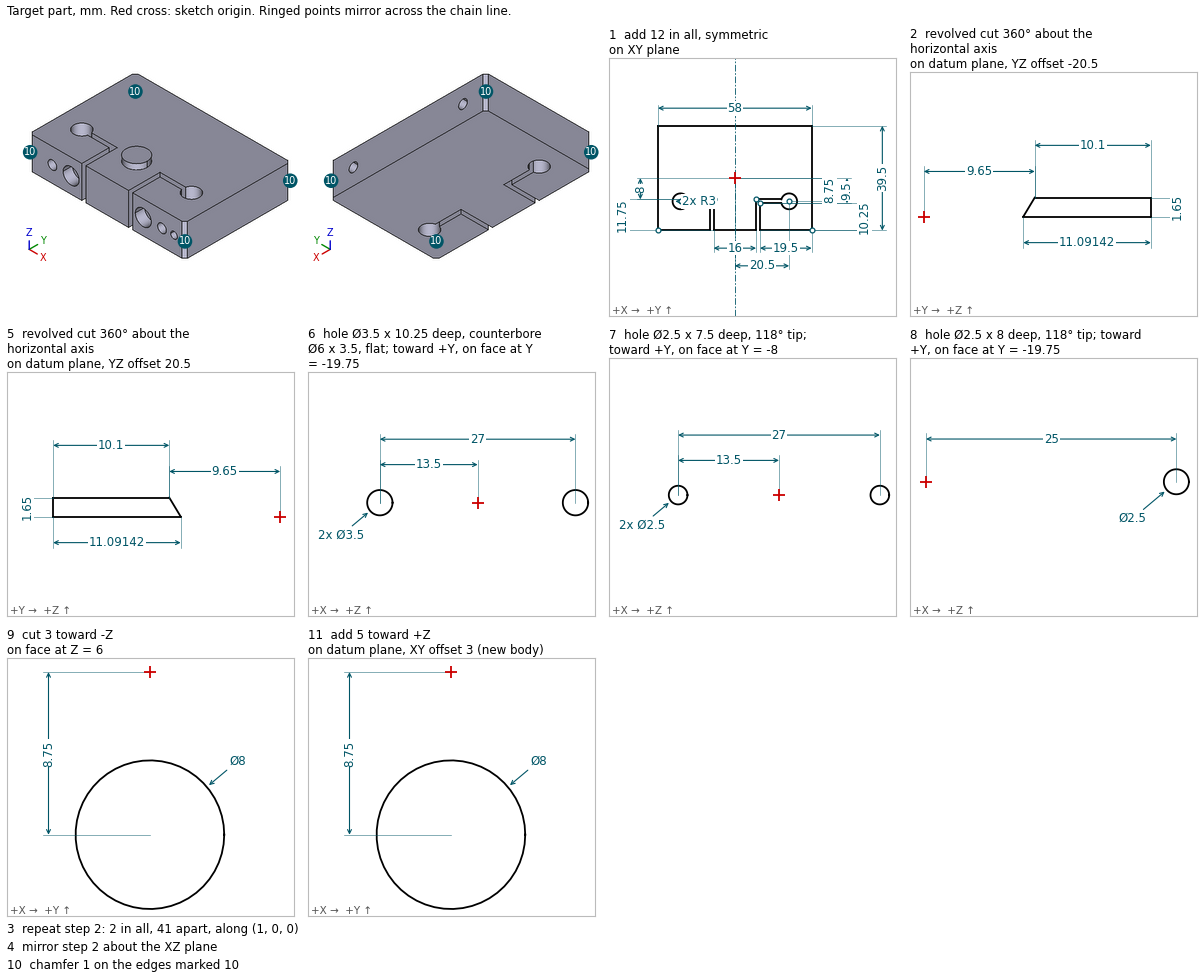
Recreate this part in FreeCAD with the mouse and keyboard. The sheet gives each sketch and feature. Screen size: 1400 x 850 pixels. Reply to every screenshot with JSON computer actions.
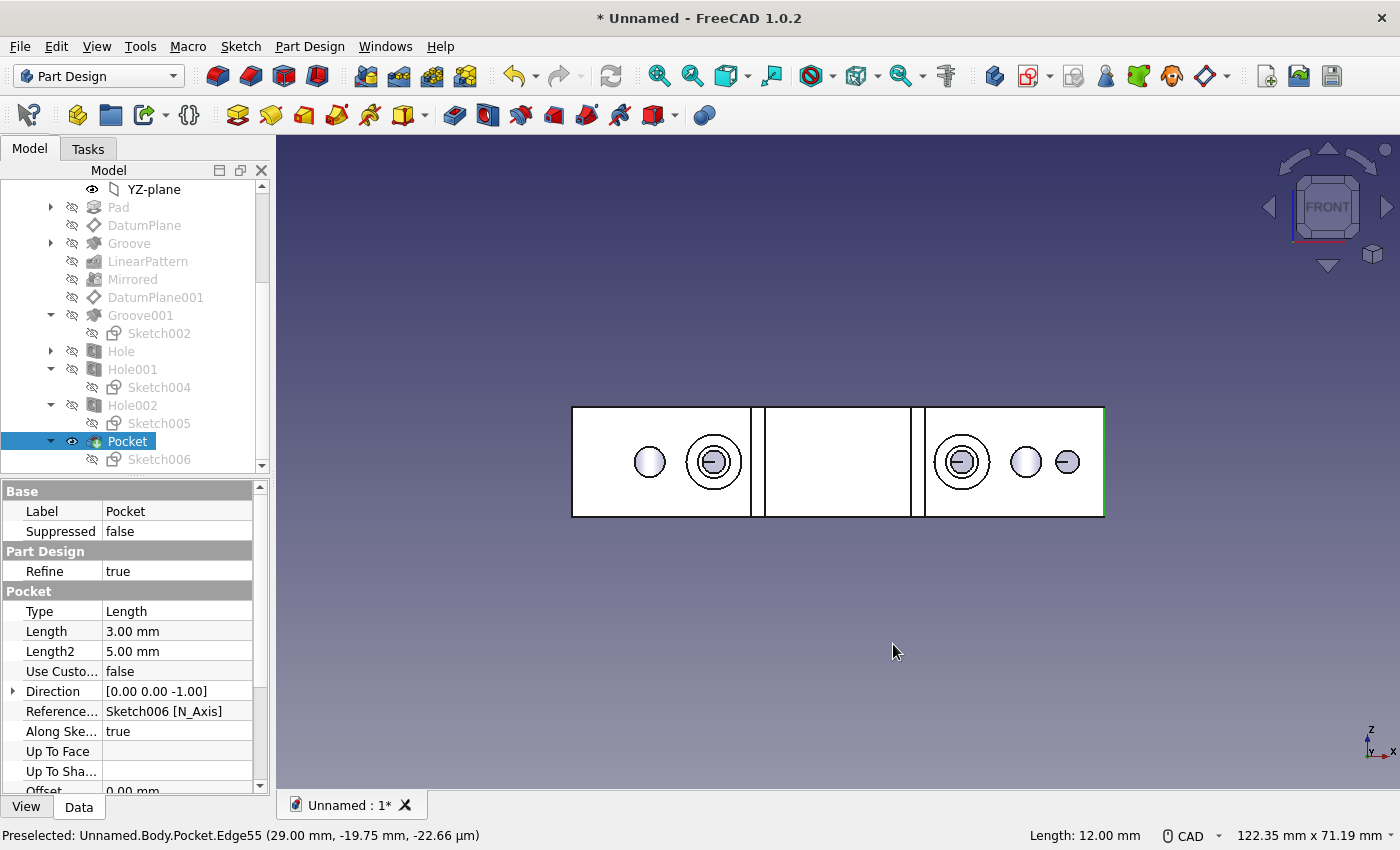
{"action": "left_click", "coordinate": [572, 461], "text": "ctrl"}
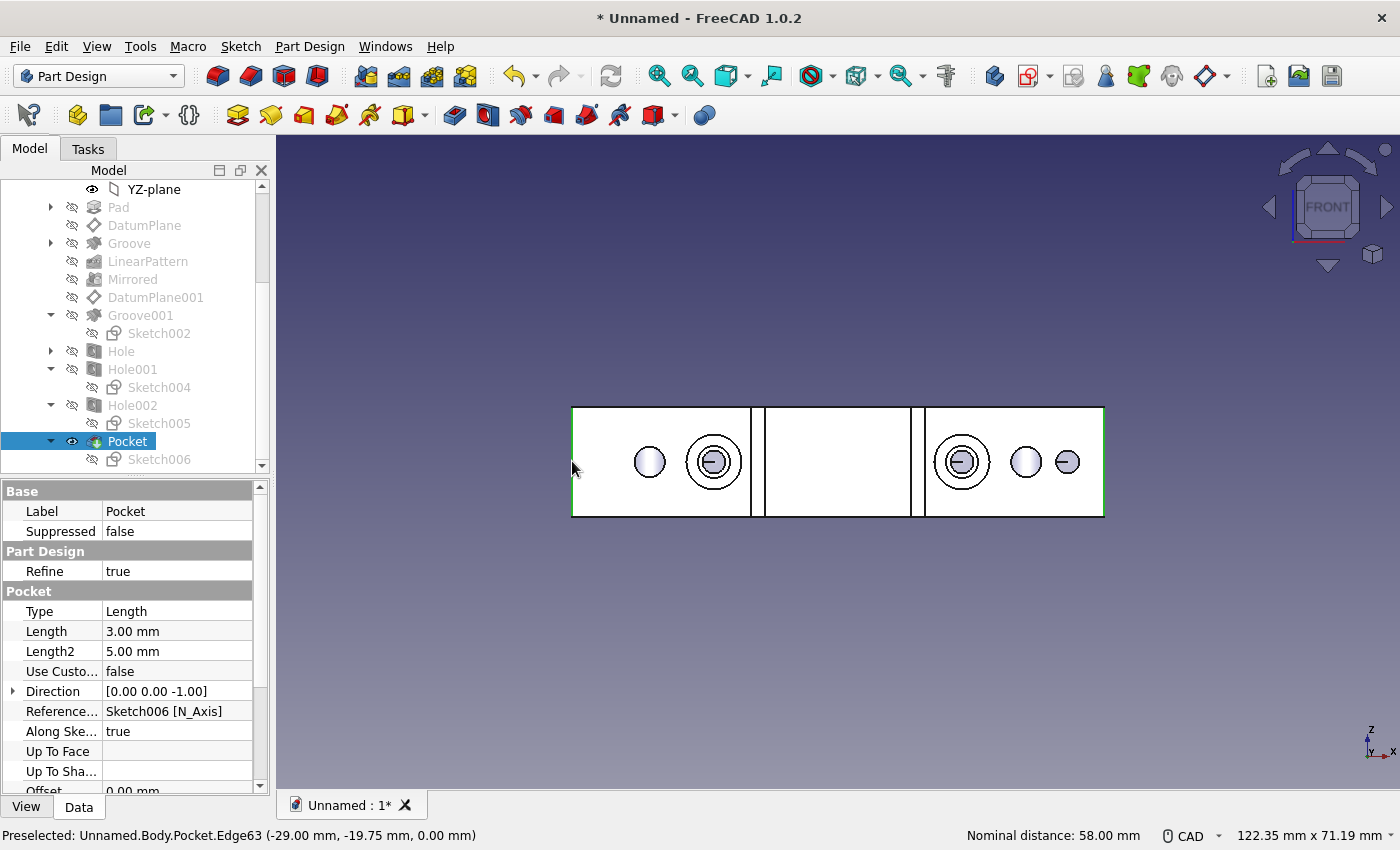
{"action": "key", "text": "3"}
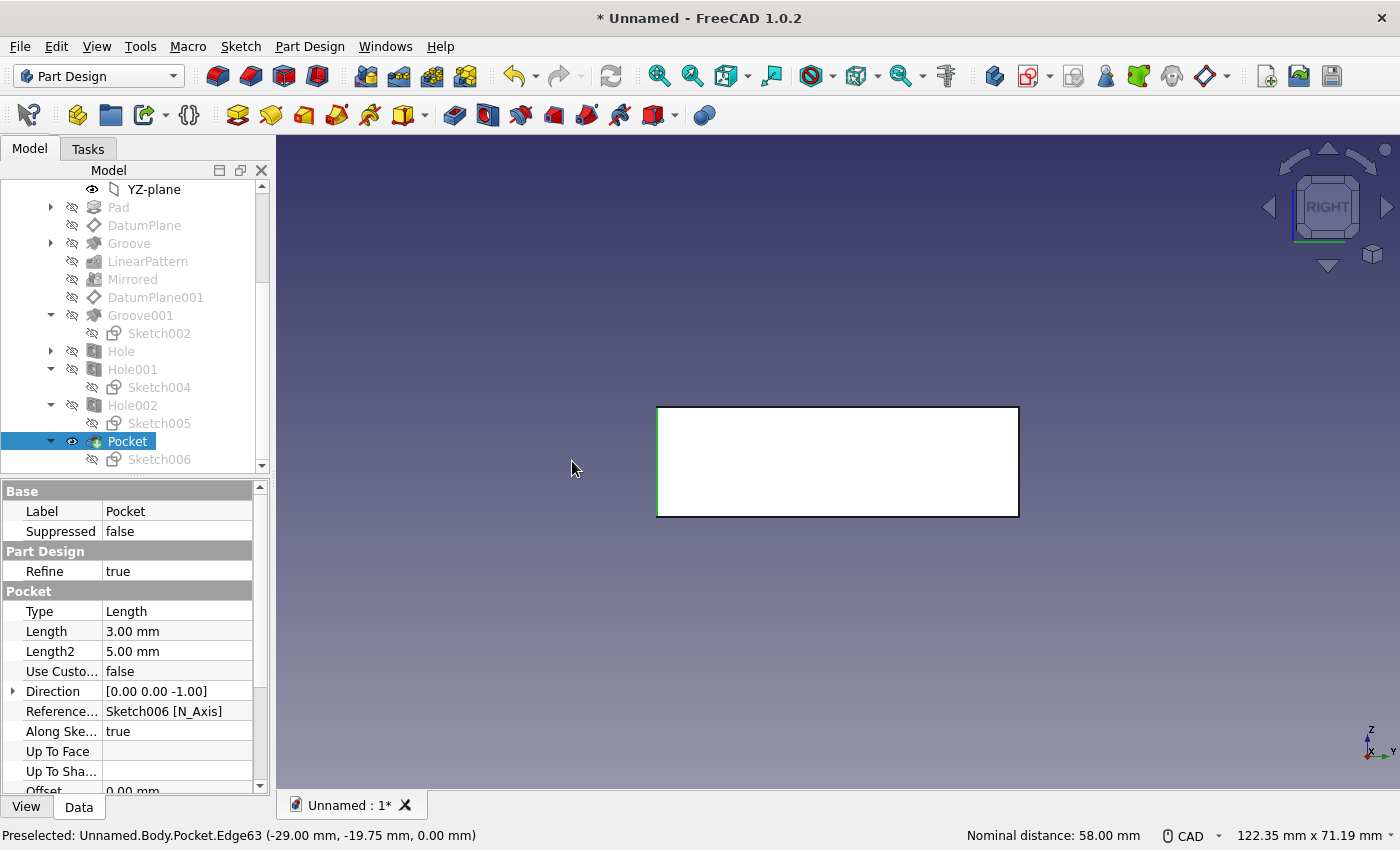
{"action": "left_click", "coordinate": [660, 76]}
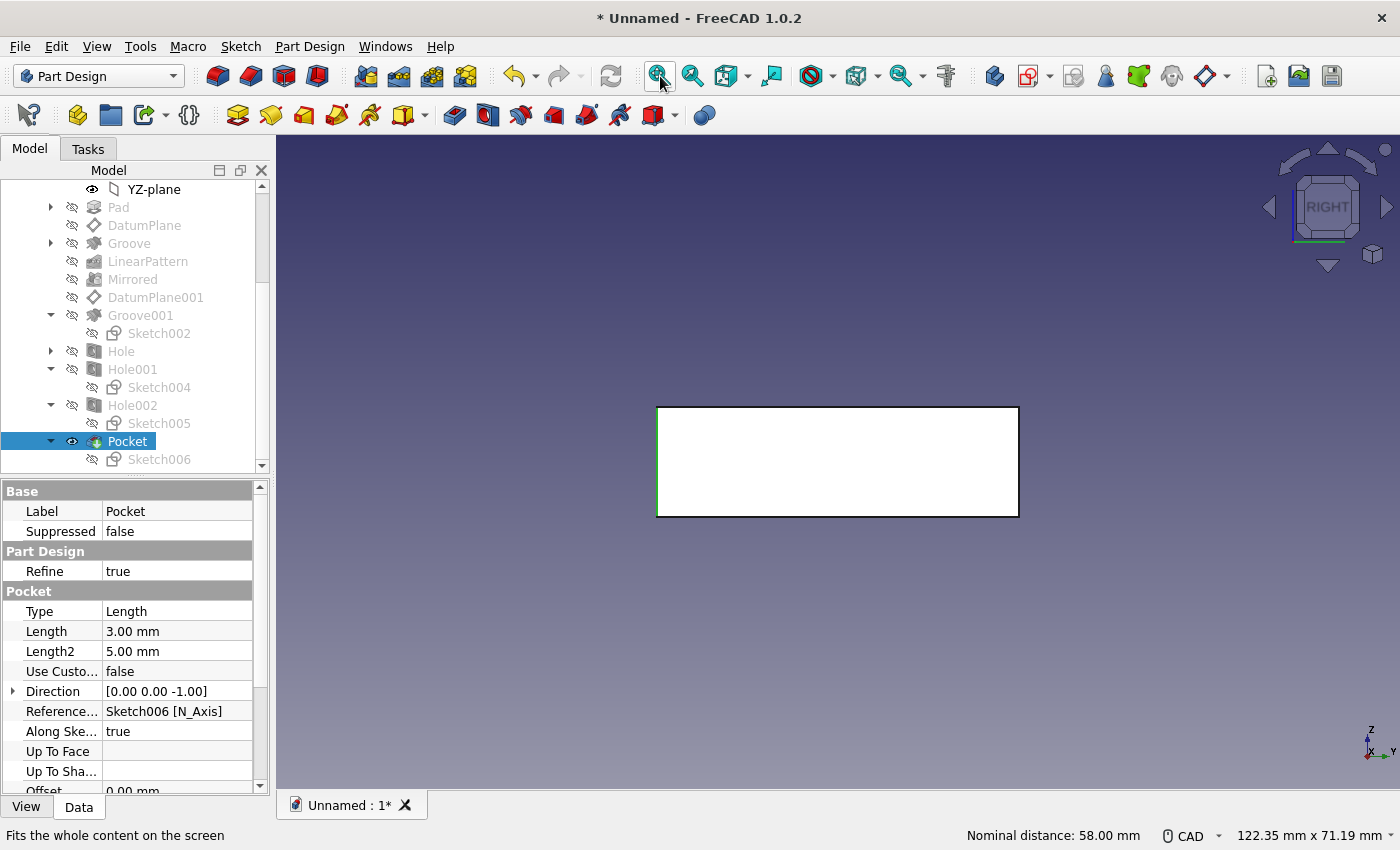
{"action": "left_click", "coordinate": [1019, 461], "text": "ctrl"}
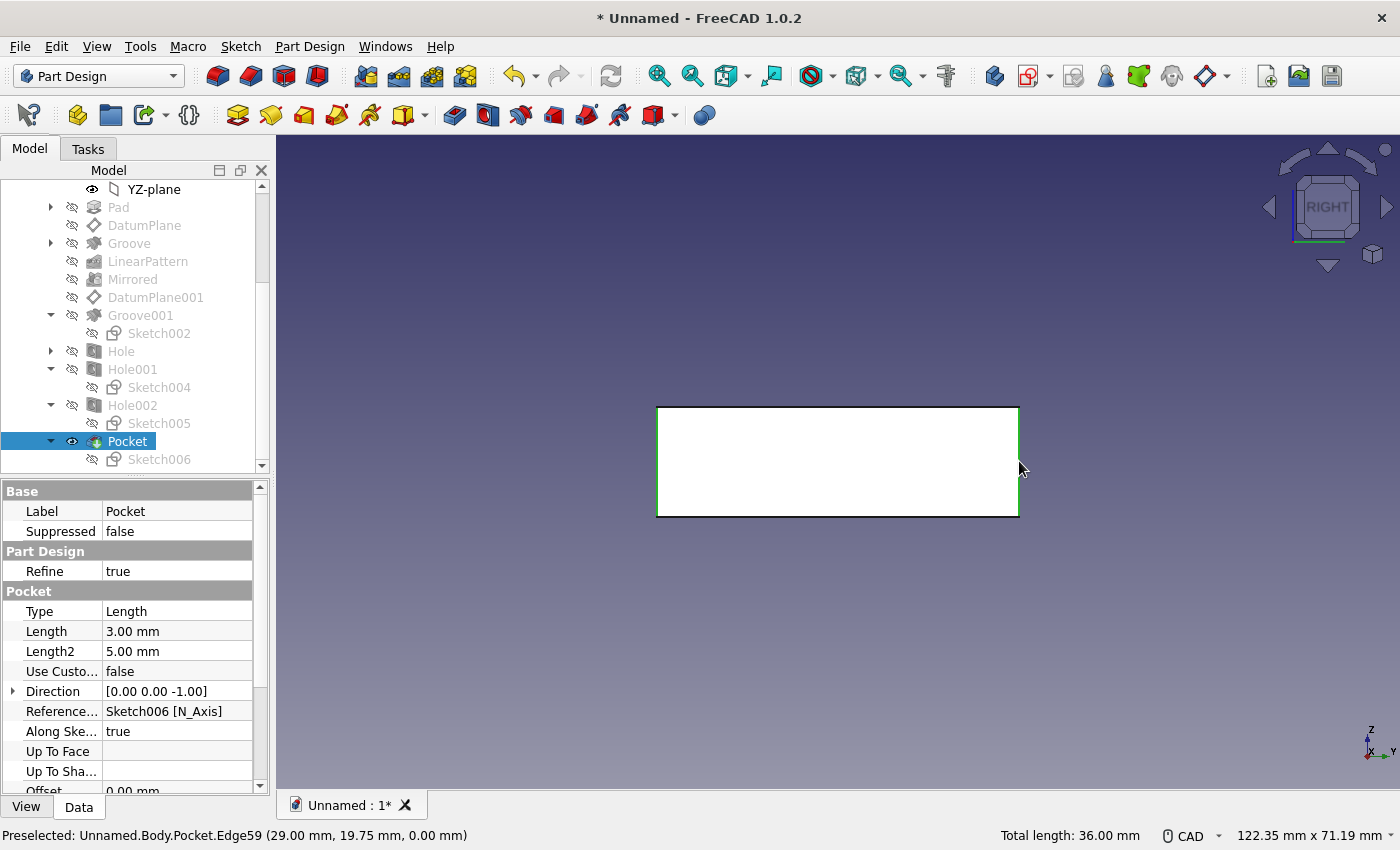
{"action": "key", "text": "5"}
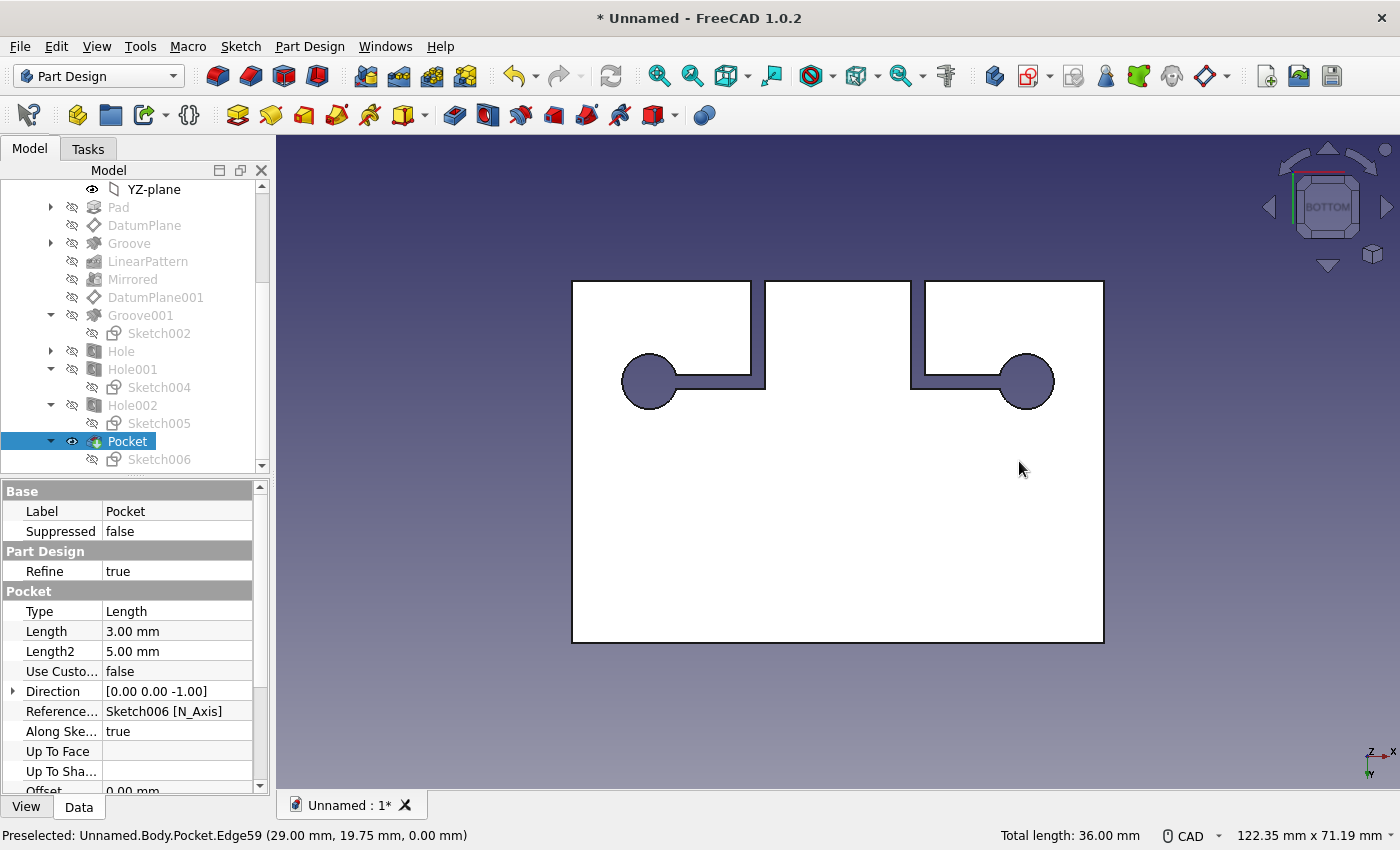
{"action": "key", "text": "4"}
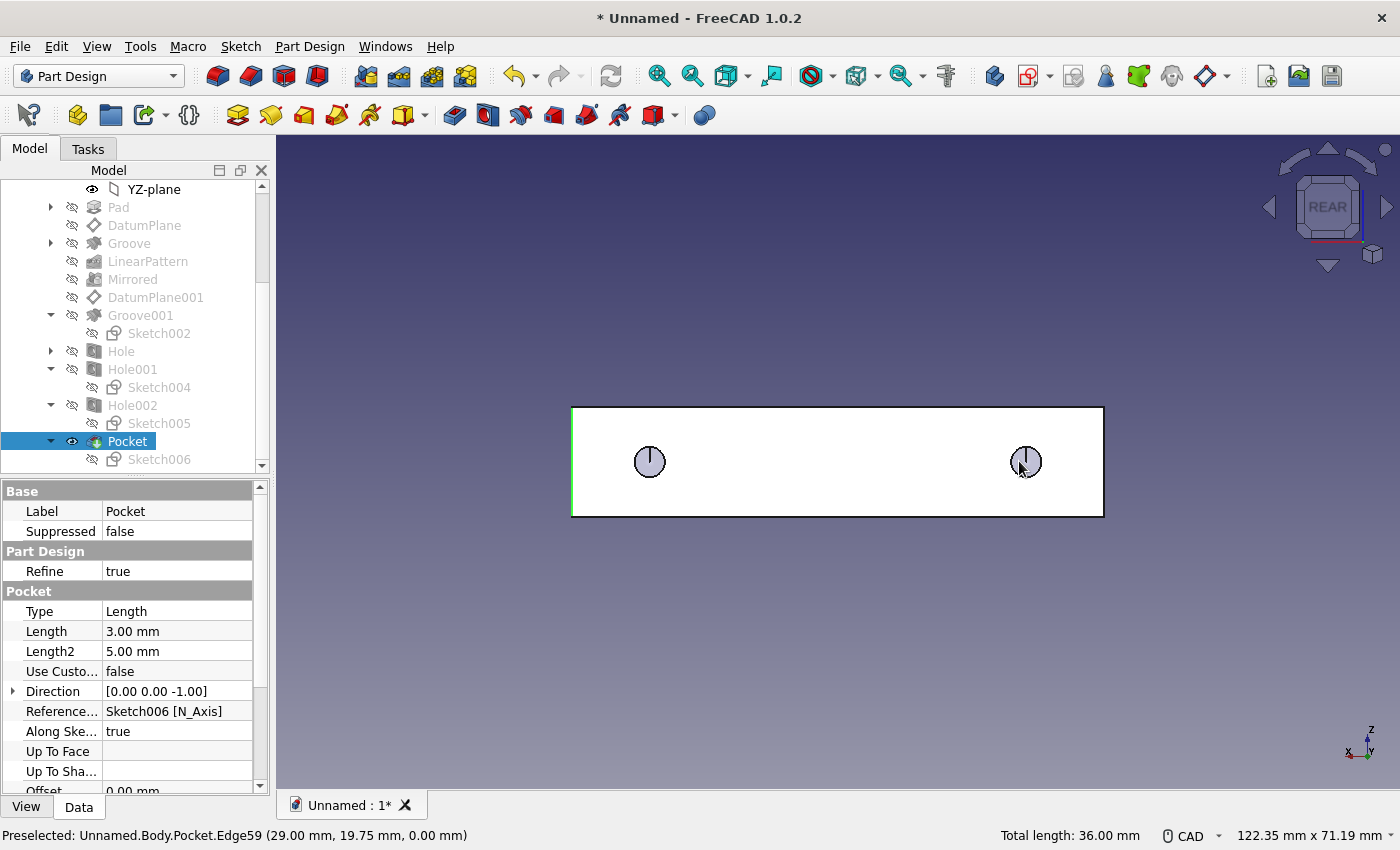
{"action": "left_click", "coordinate": [1104, 461], "text": "ctrl"}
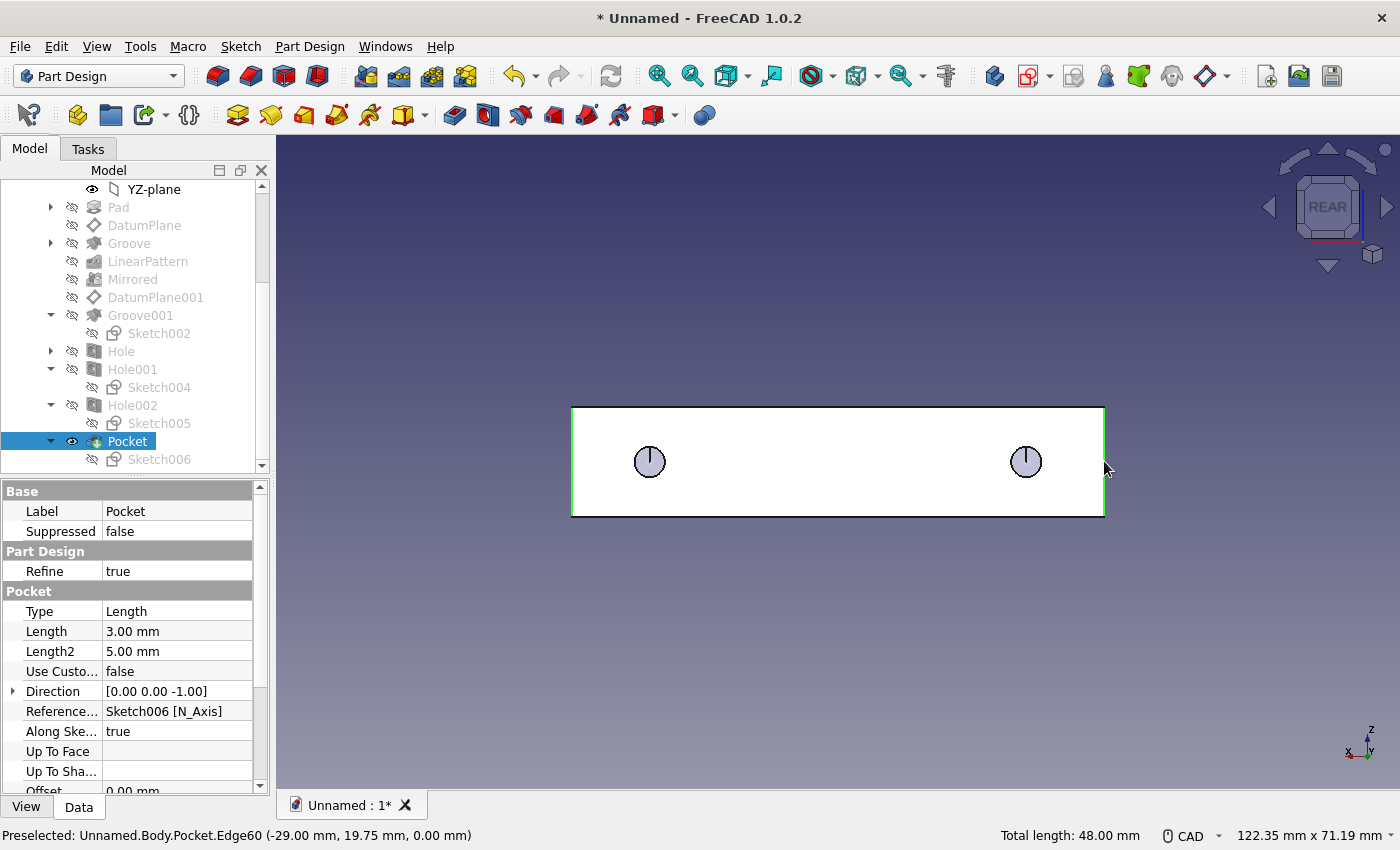
{"action": "left_click", "coordinate": [251, 76]}